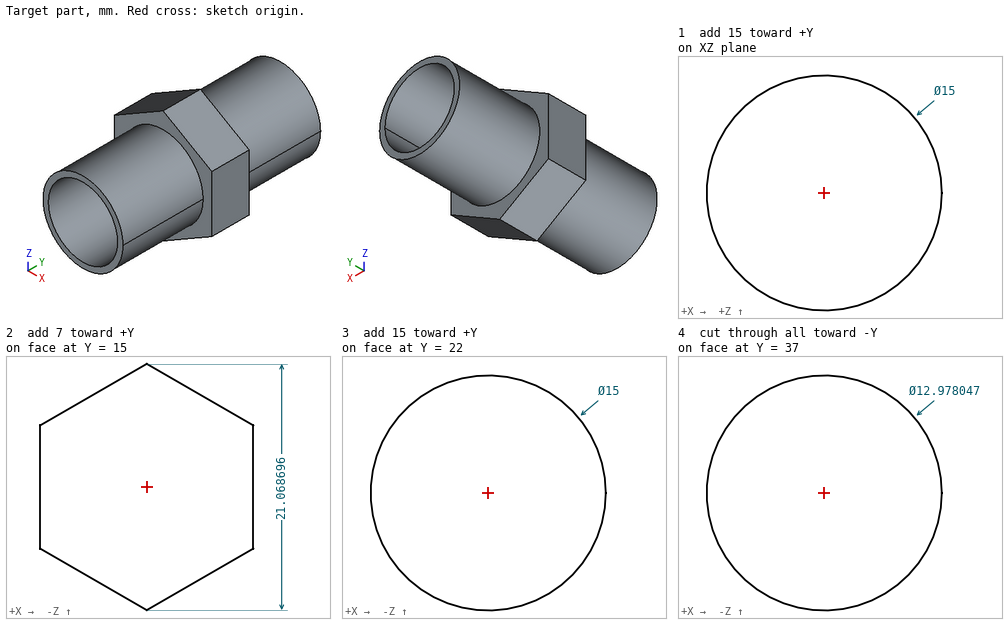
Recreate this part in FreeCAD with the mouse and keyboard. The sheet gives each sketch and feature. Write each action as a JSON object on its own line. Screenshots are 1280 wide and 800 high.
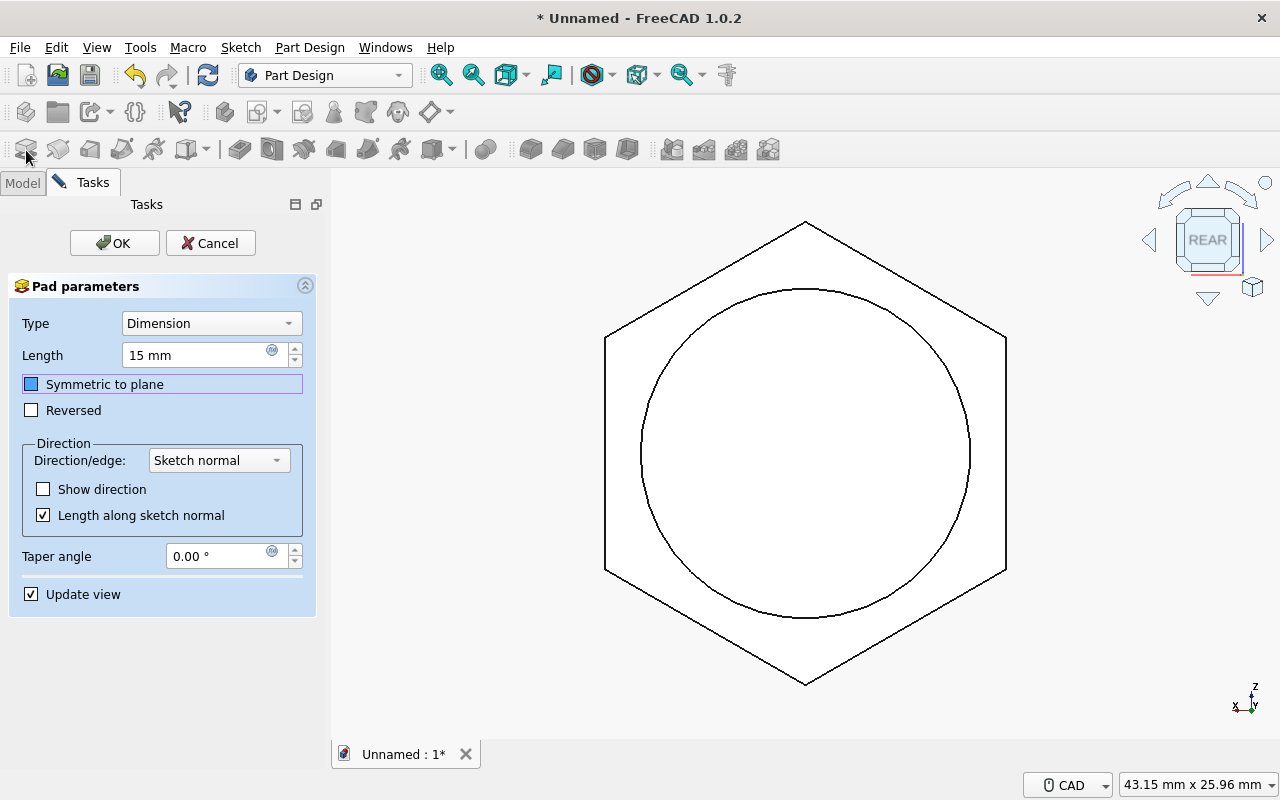
{"action": "left_click", "coordinate": [115, 243]}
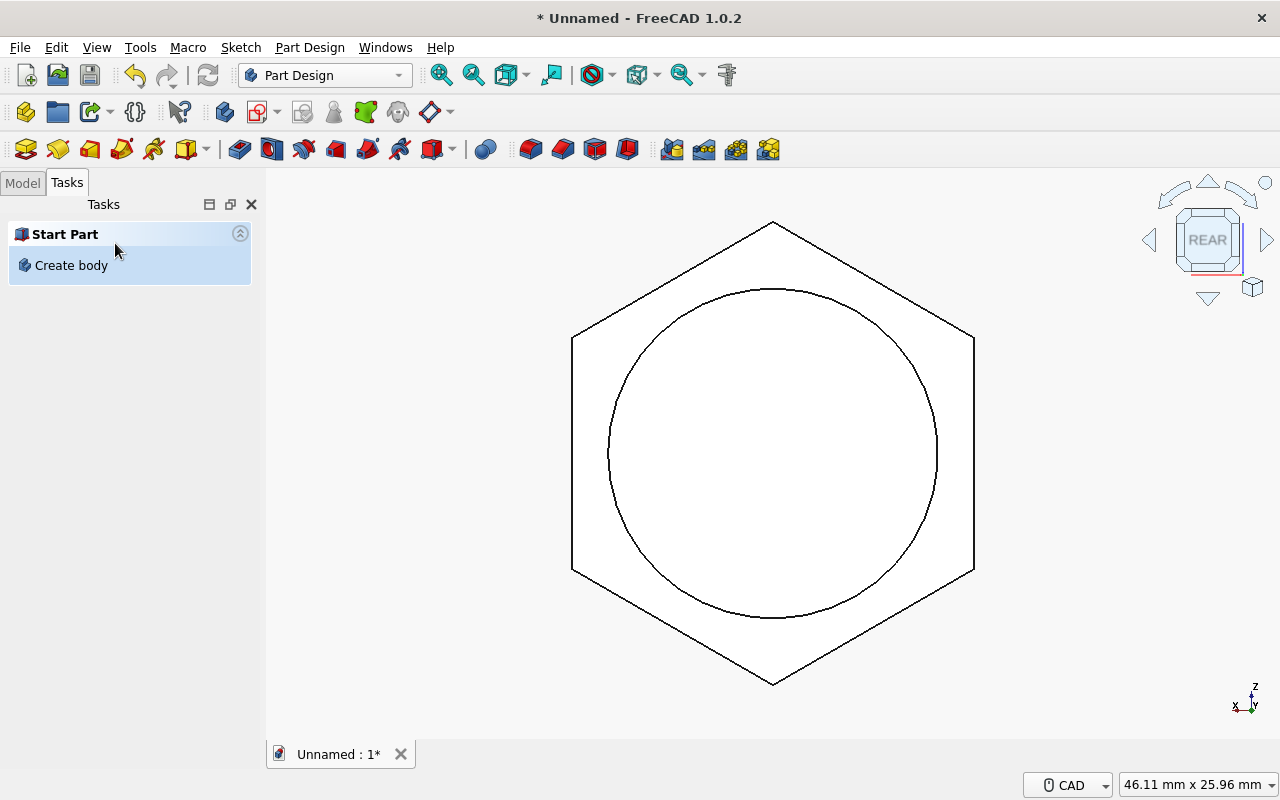
{"action": "left_click", "coordinate": [773, 453]}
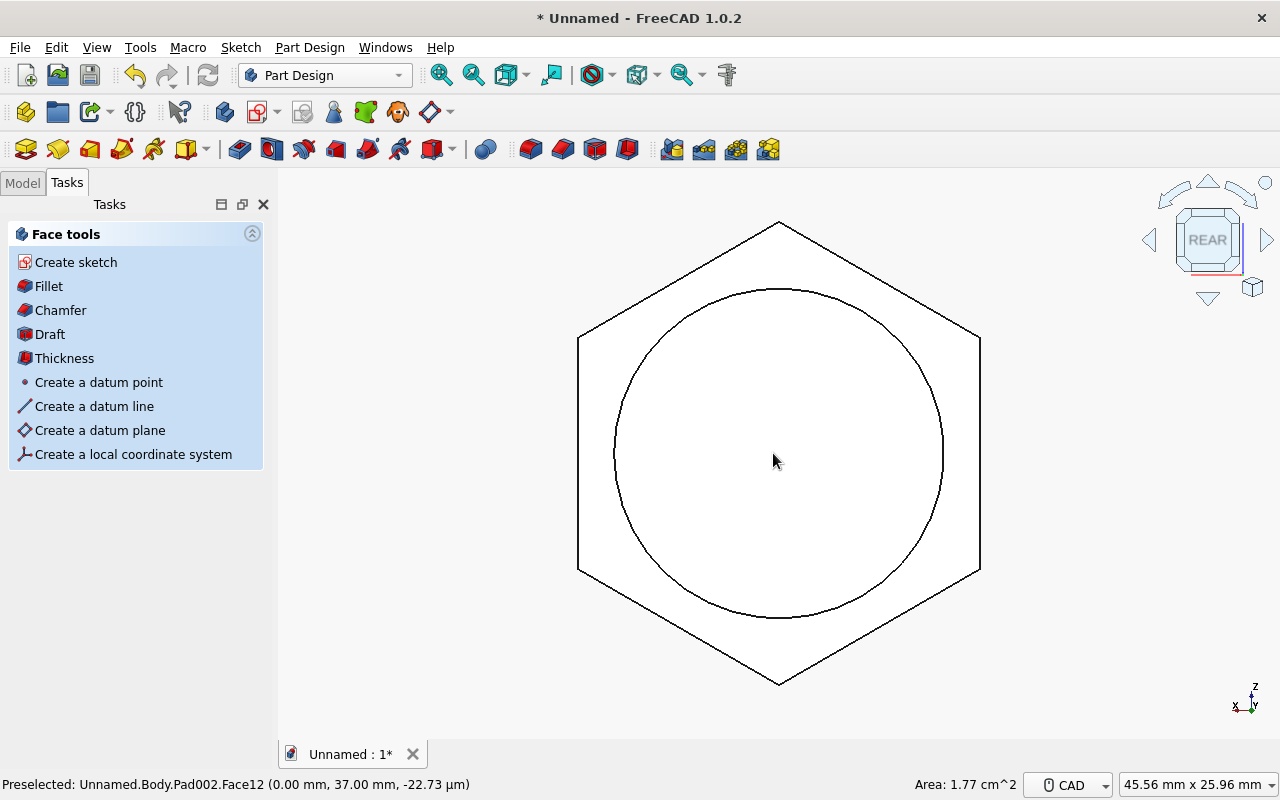
{"action": "left_click", "coordinate": [258, 112]}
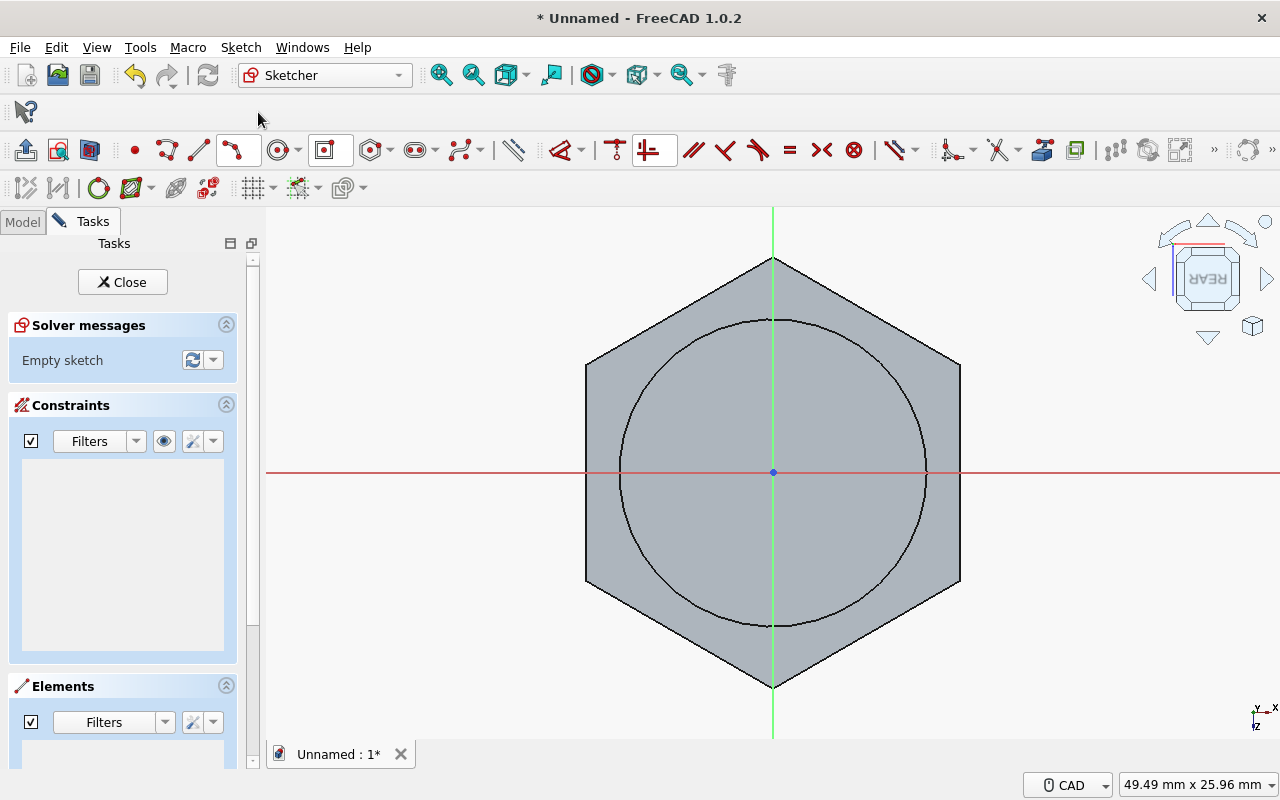
{"action": "left_click", "coordinate": [278, 150]}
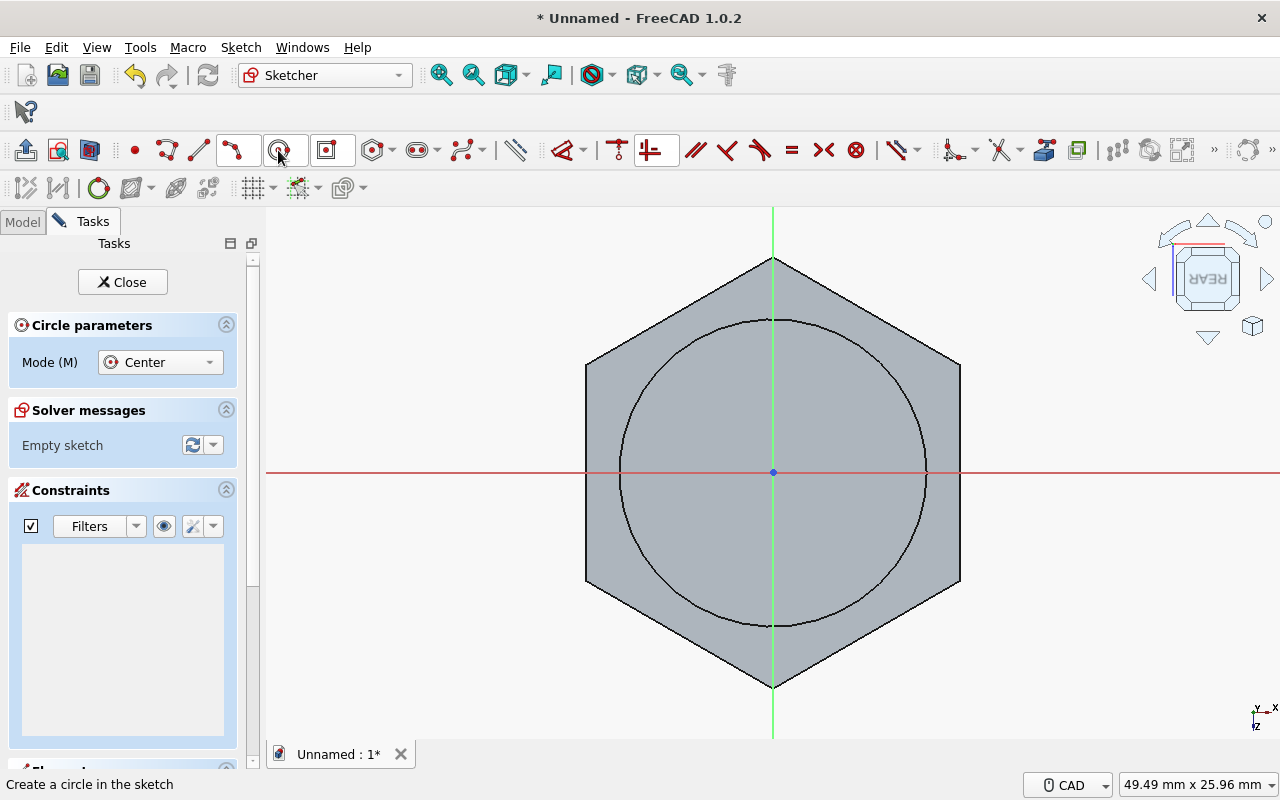
{"action": "left_click", "coordinate": [773, 473]}
{"action": "mouse_move", "coordinate": [867, 379]}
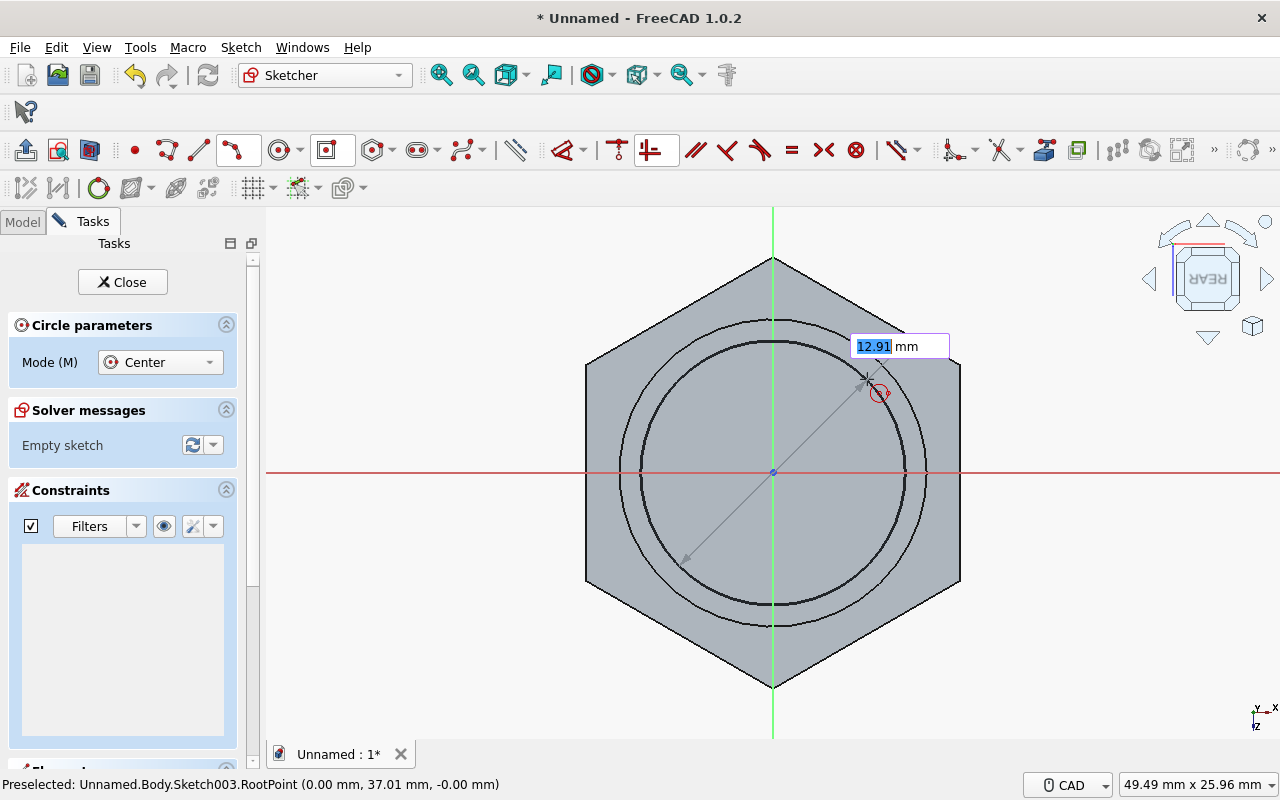
{"action": "type", "text": "12.978047"}
{"action": "key", "text": "Return"}
{"action": "key", "text": "Escape"}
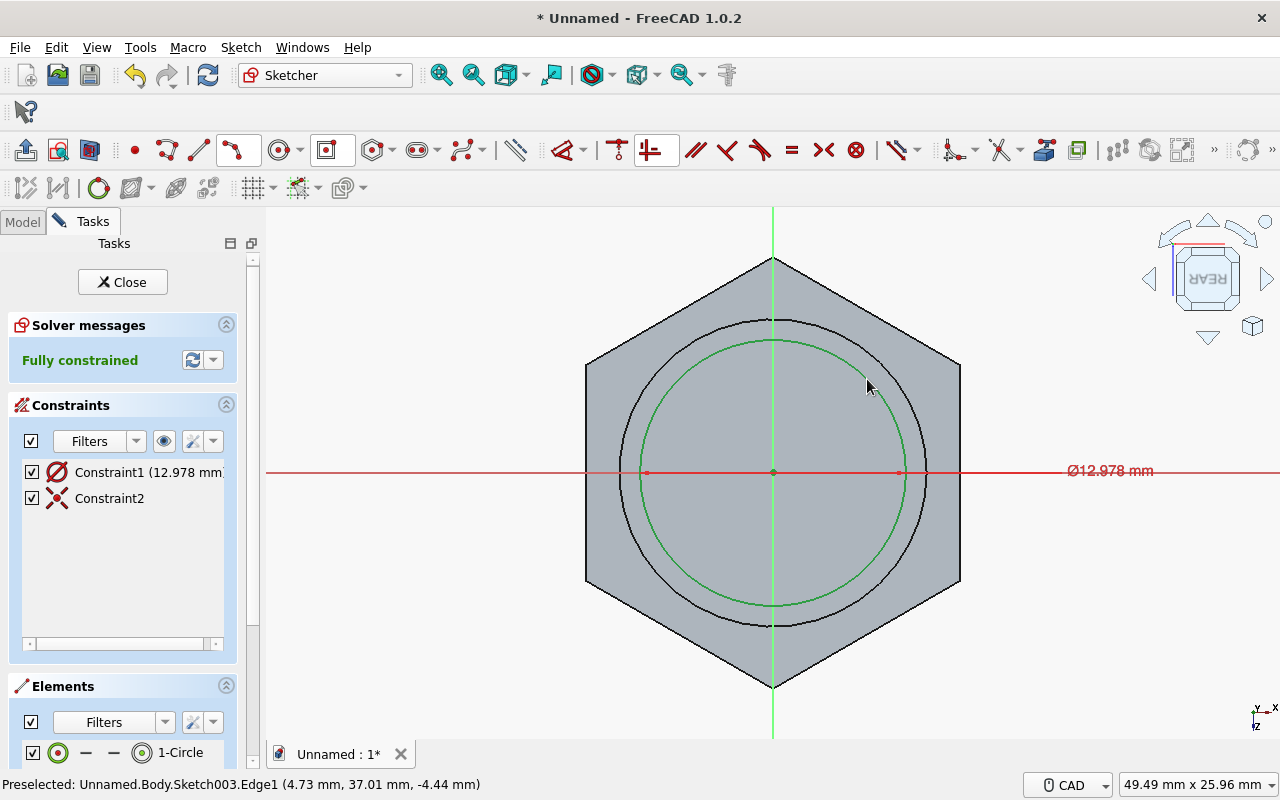
{"action": "left_click", "coordinate": [123, 282]}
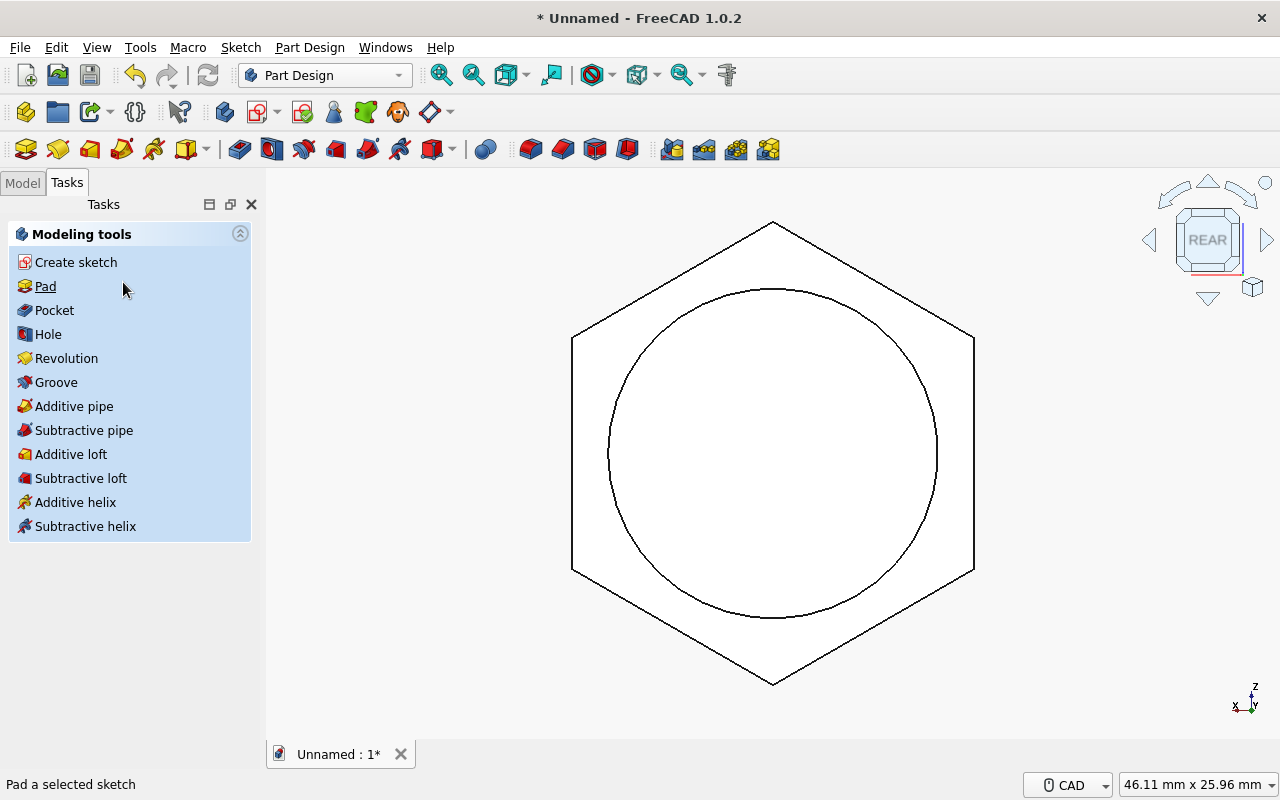
{"action": "left_click", "coordinate": [240, 150]}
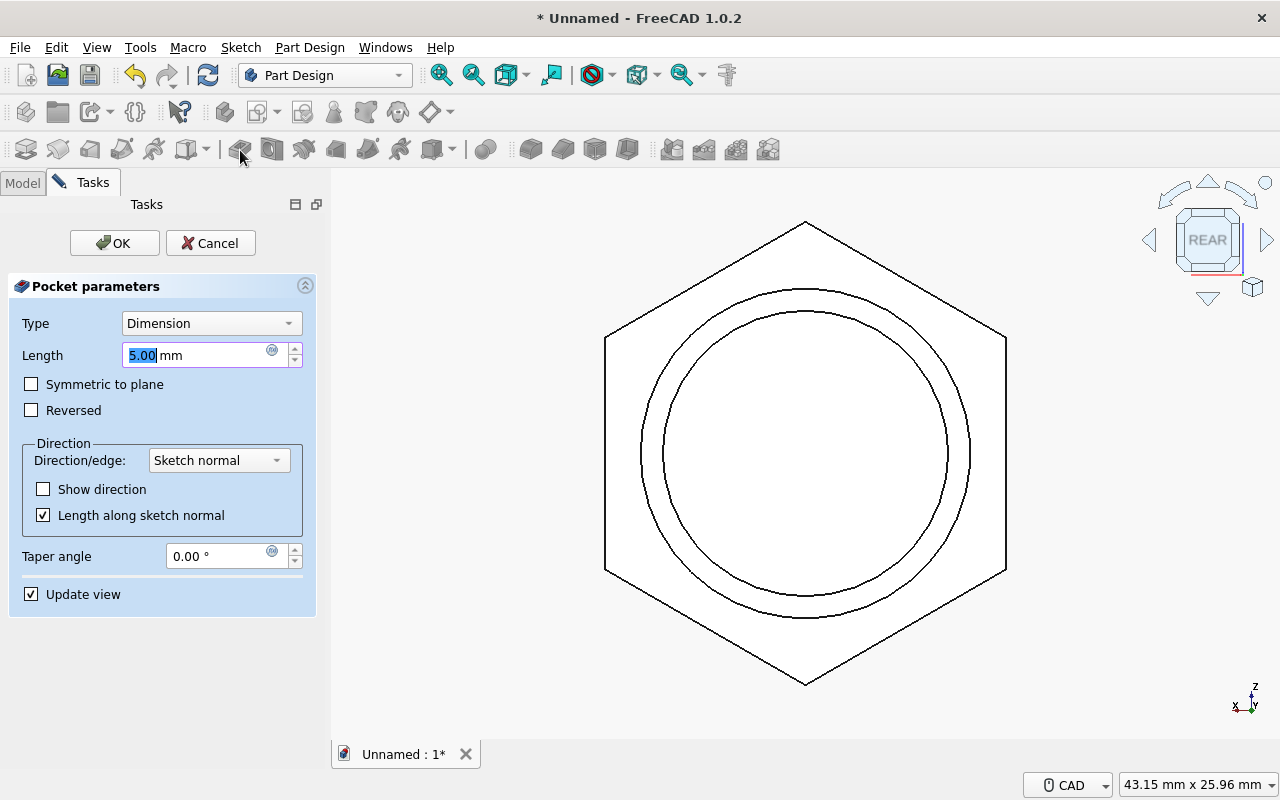
{"action": "left_click", "coordinate": [212, 324]}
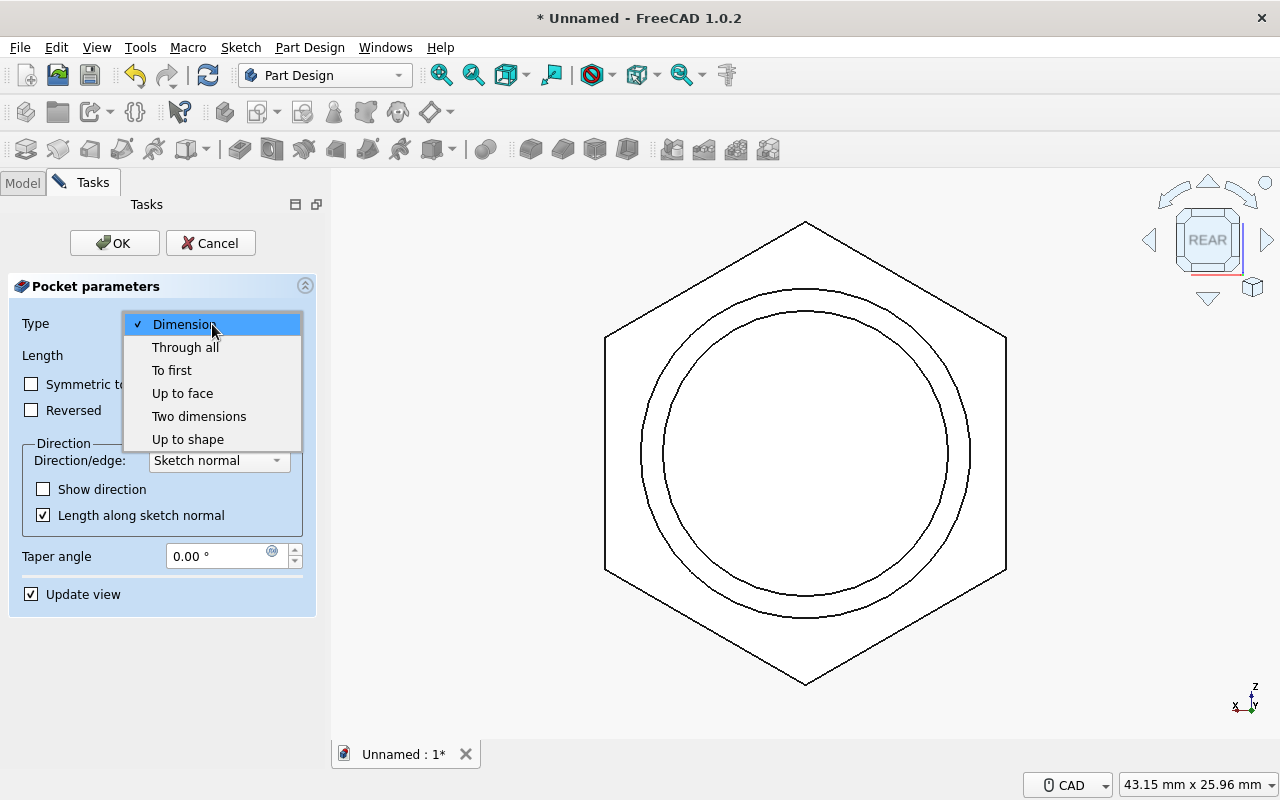
{"action": "left_click", "coordinate": [212, 348]}